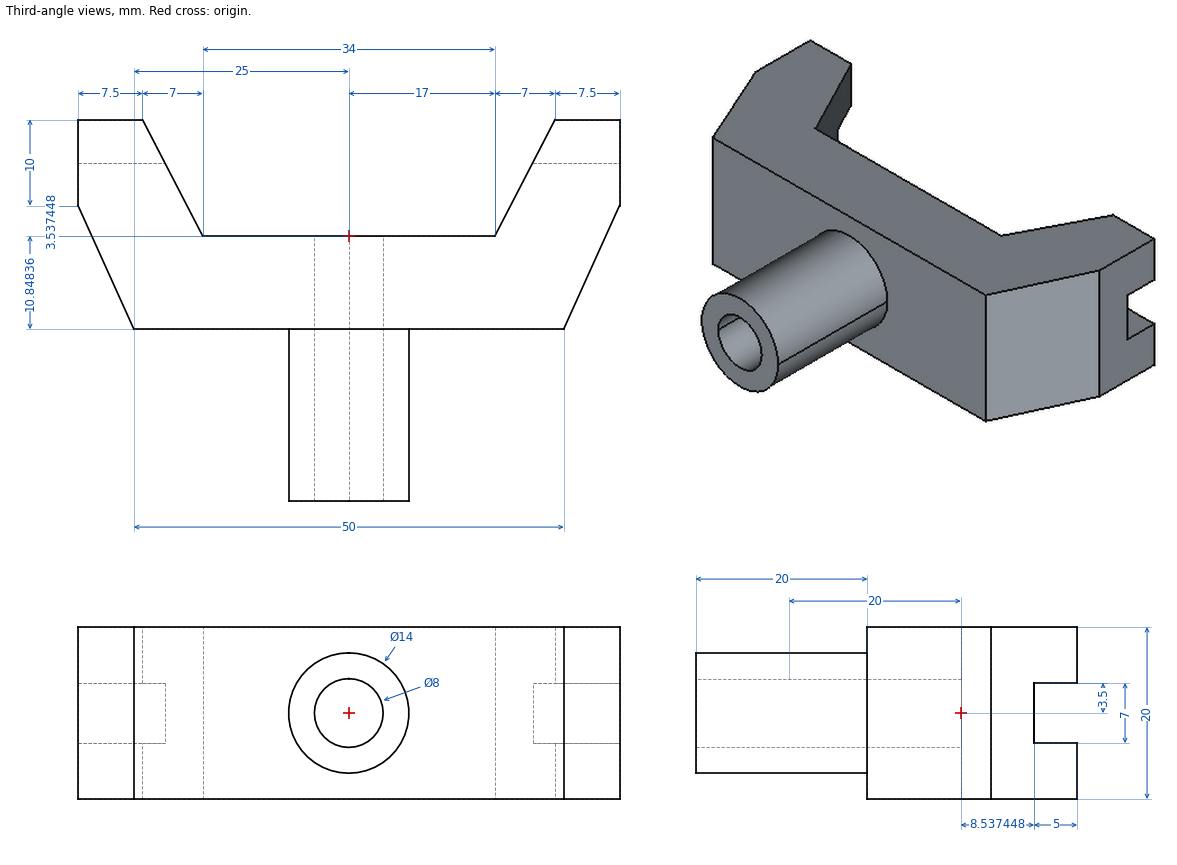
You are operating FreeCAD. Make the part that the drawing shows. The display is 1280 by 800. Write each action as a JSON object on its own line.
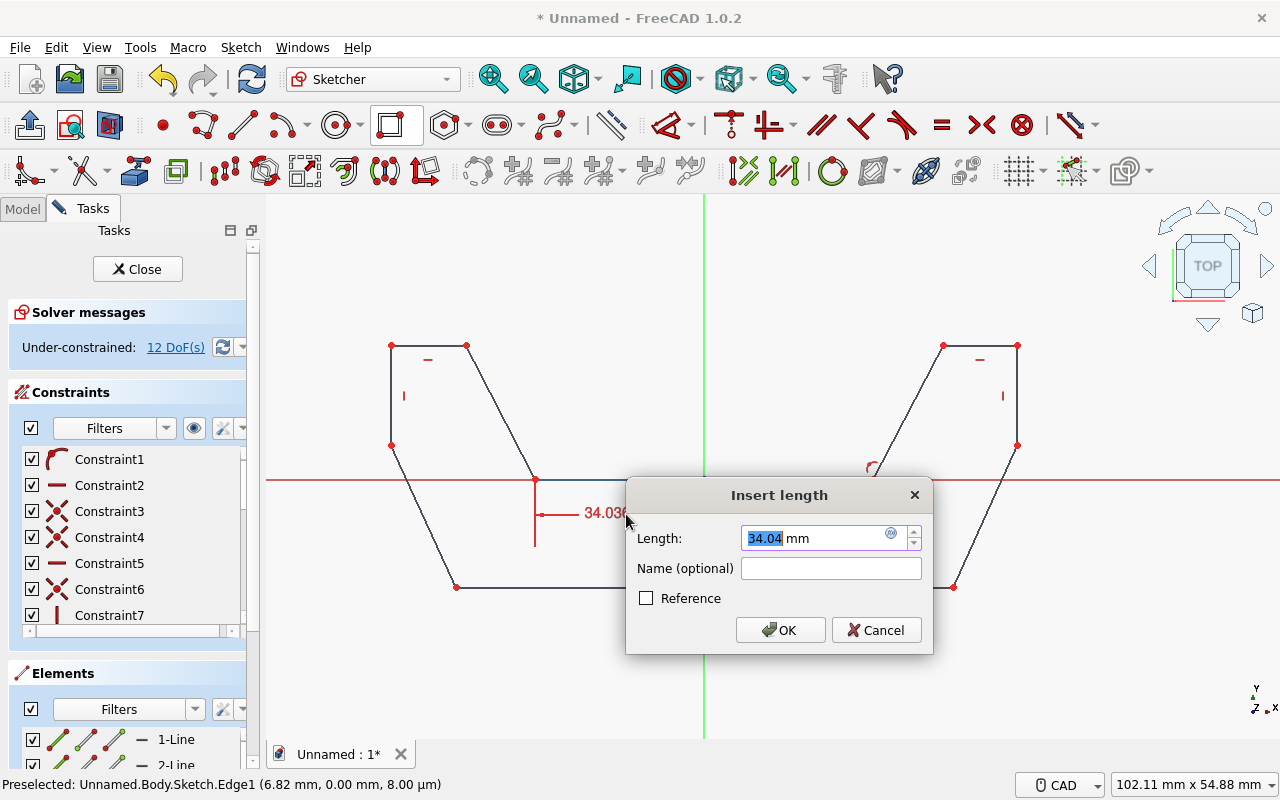
{"action": "type", "text": "34"}
{"action": "key", "text": "Return"}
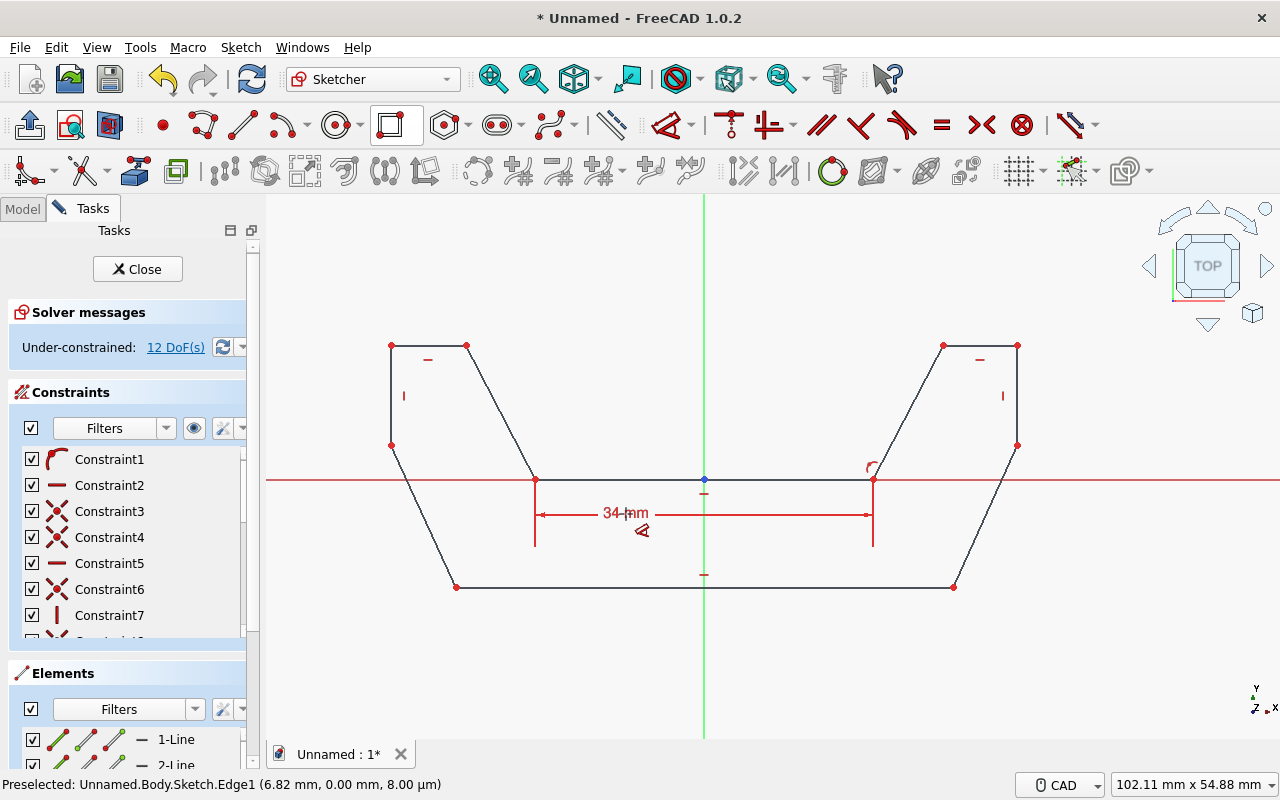
{"action": "left_click", "coordinate": [391, 376]}
{"action": "left_click", "coordinate": [357, 396]}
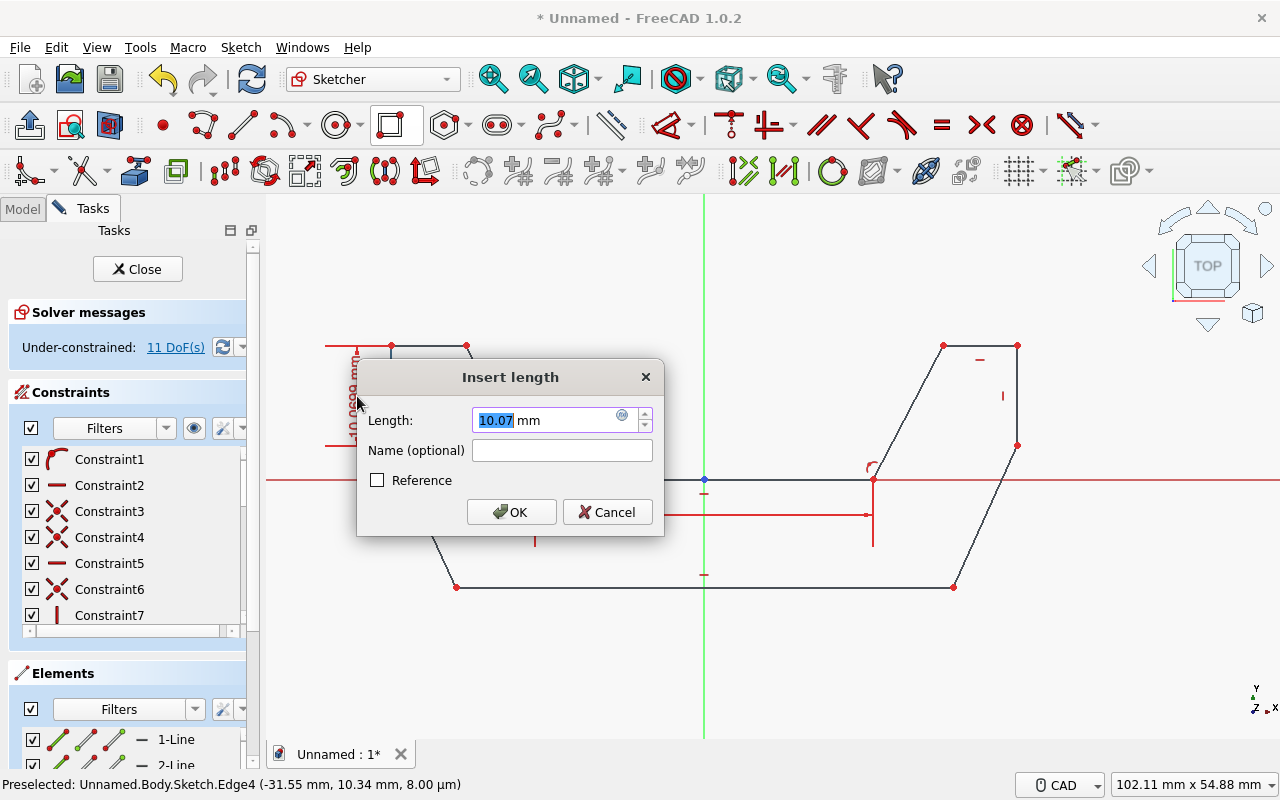
{"action": "type", "text": "10"}
{"action": "key", "text": "Return"}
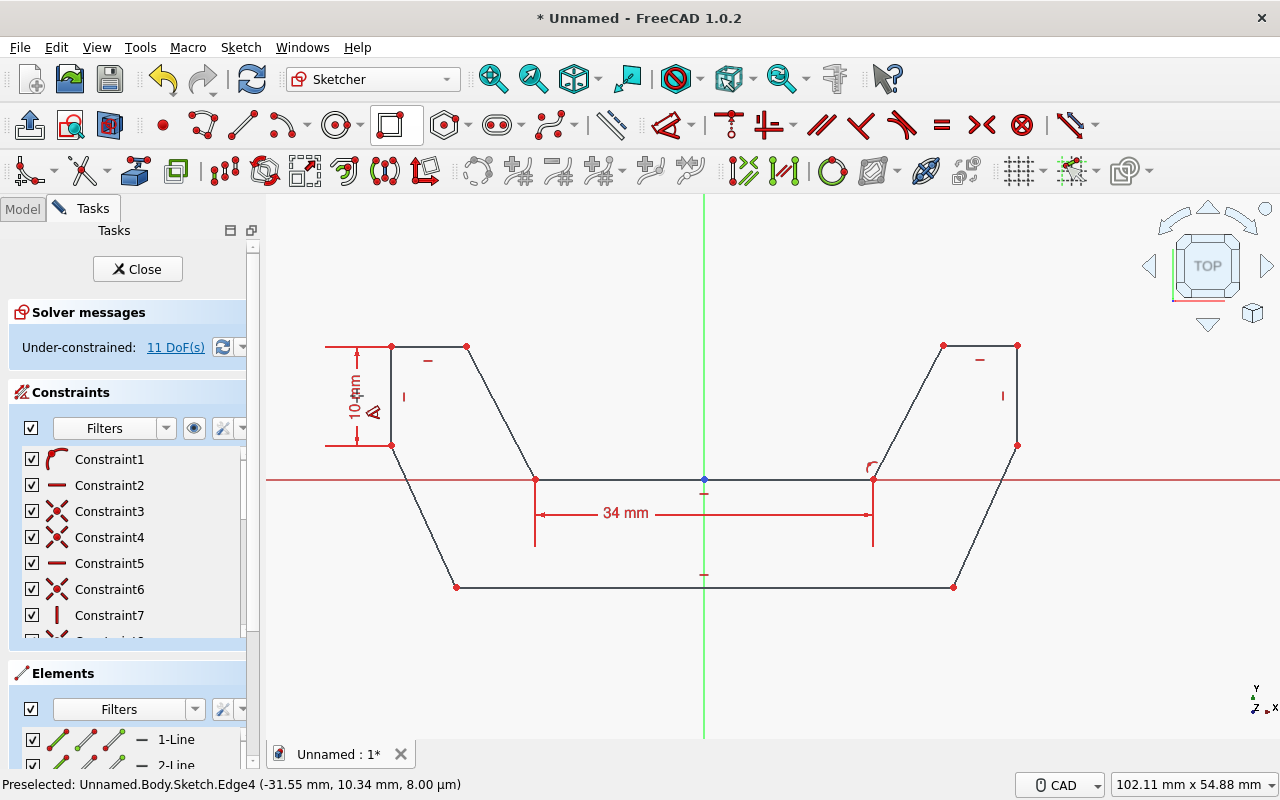
{"action": "left_click", "coordinate": [605, 588]}
{"action": "left_click", "coordinate": [590, 622]}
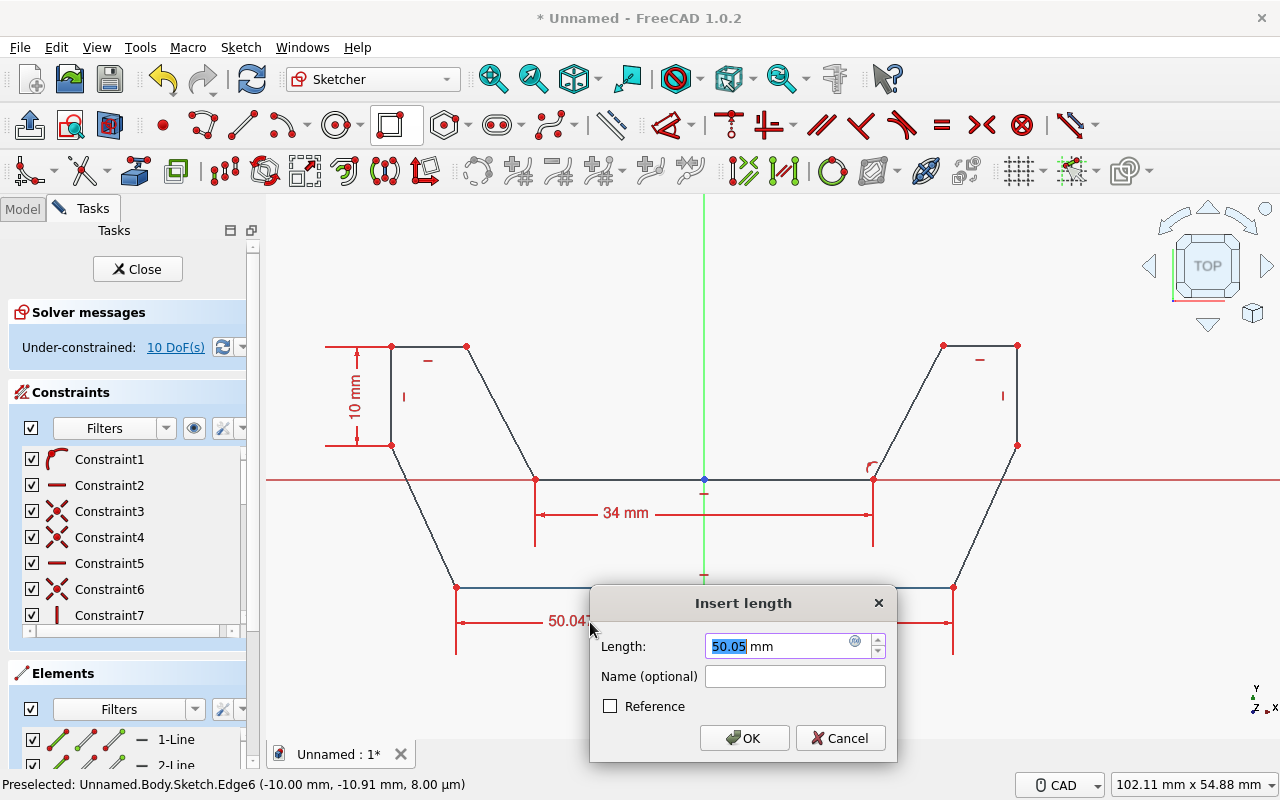
{"action": "type", "text": "50"}
{"action": "key", "text": "Return"}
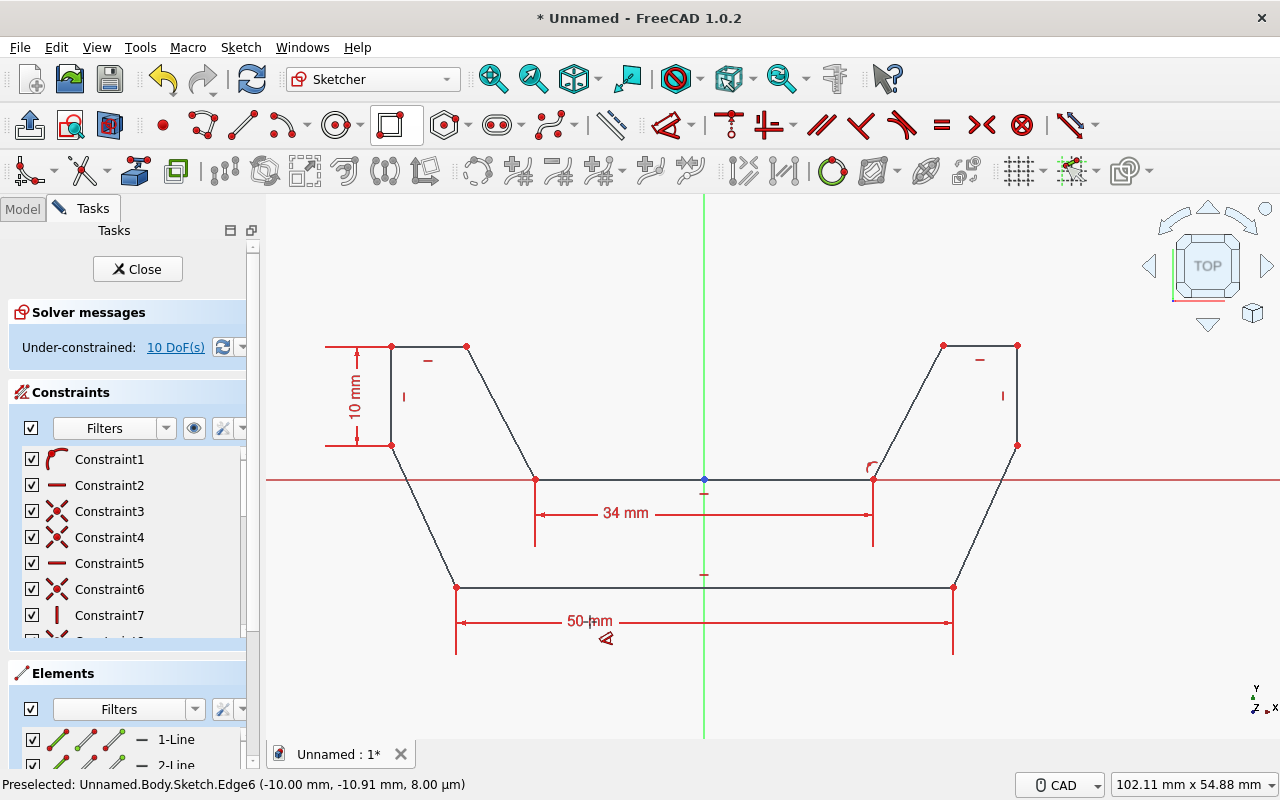
{"action": "left_click", "coordinate": [1017, 416]}
{"action": "left_click", "coordinate": [1051, 396]}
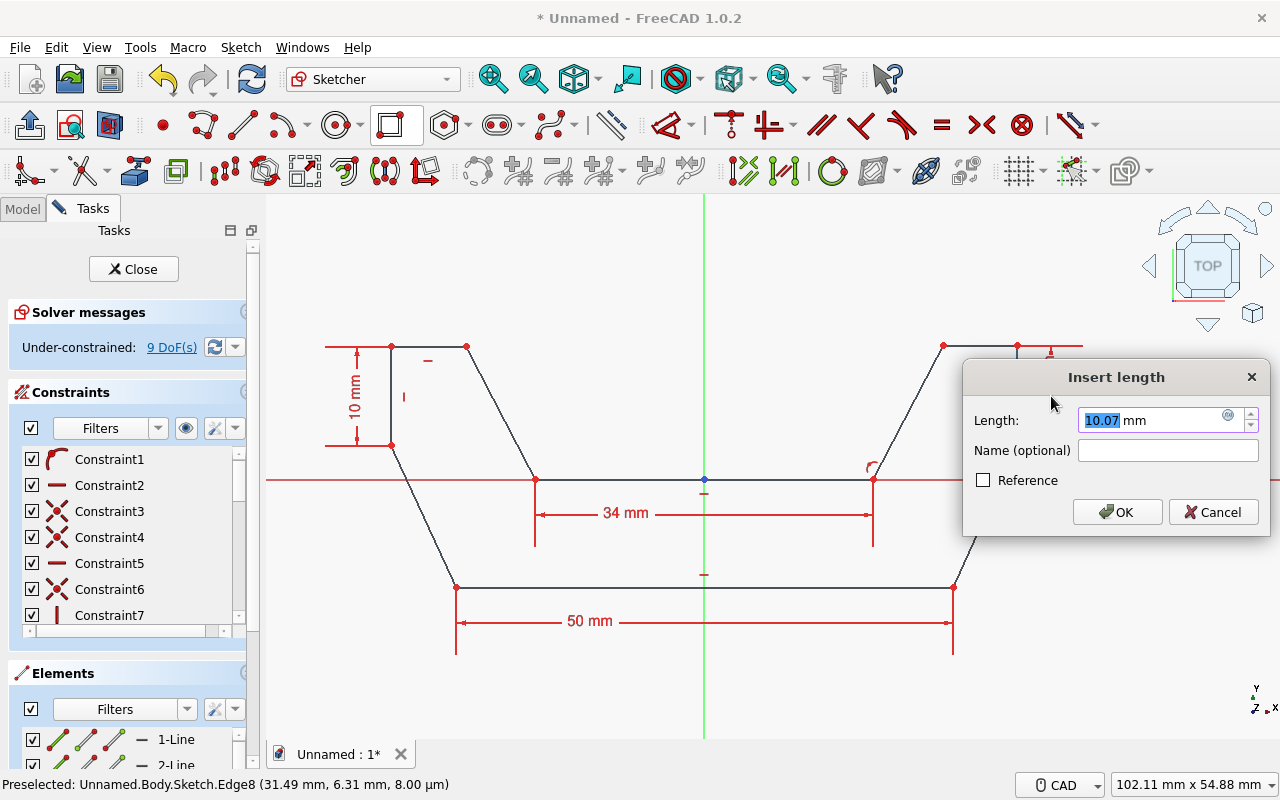
{"action": "type", "text": "10"}
{"action": "key", "text": "Return"}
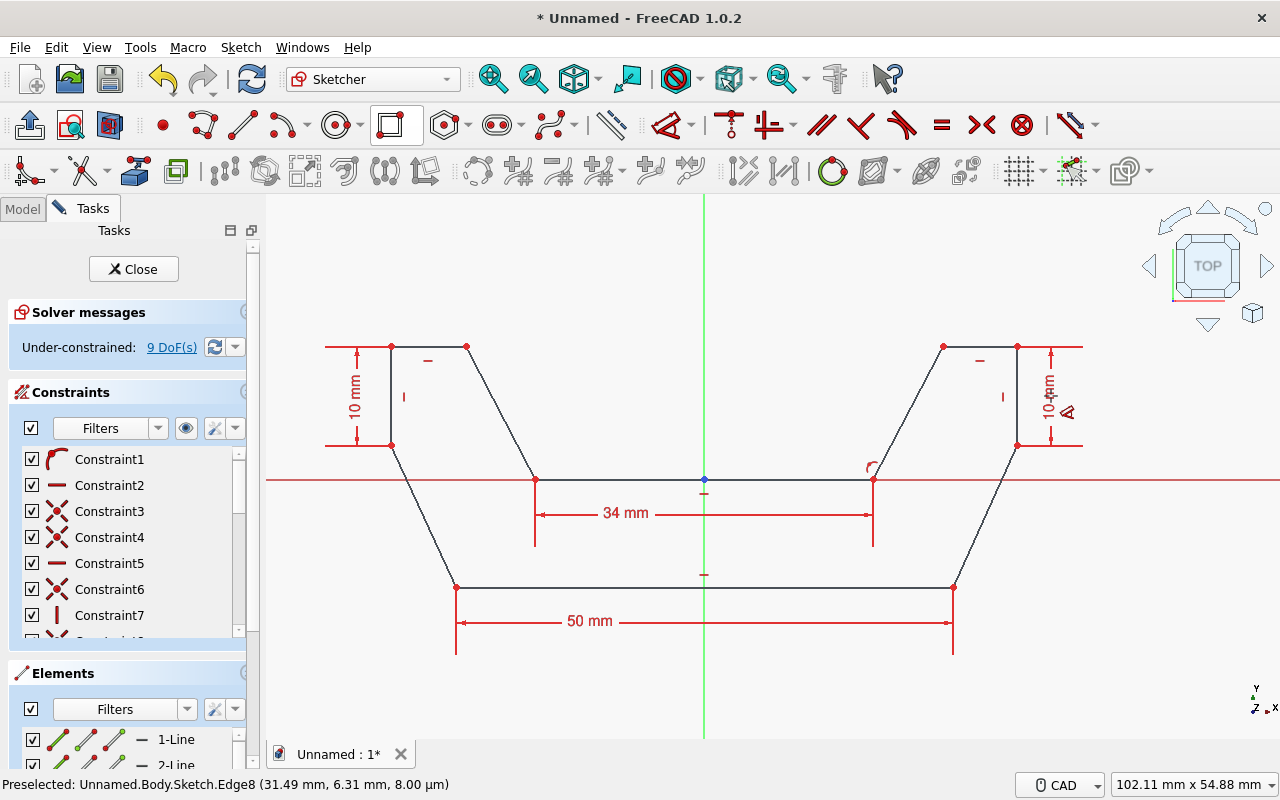
{"action": "left_click", "coordinate": [515, 440]}
{"action": "left_click", "coordinate": [501, 313]}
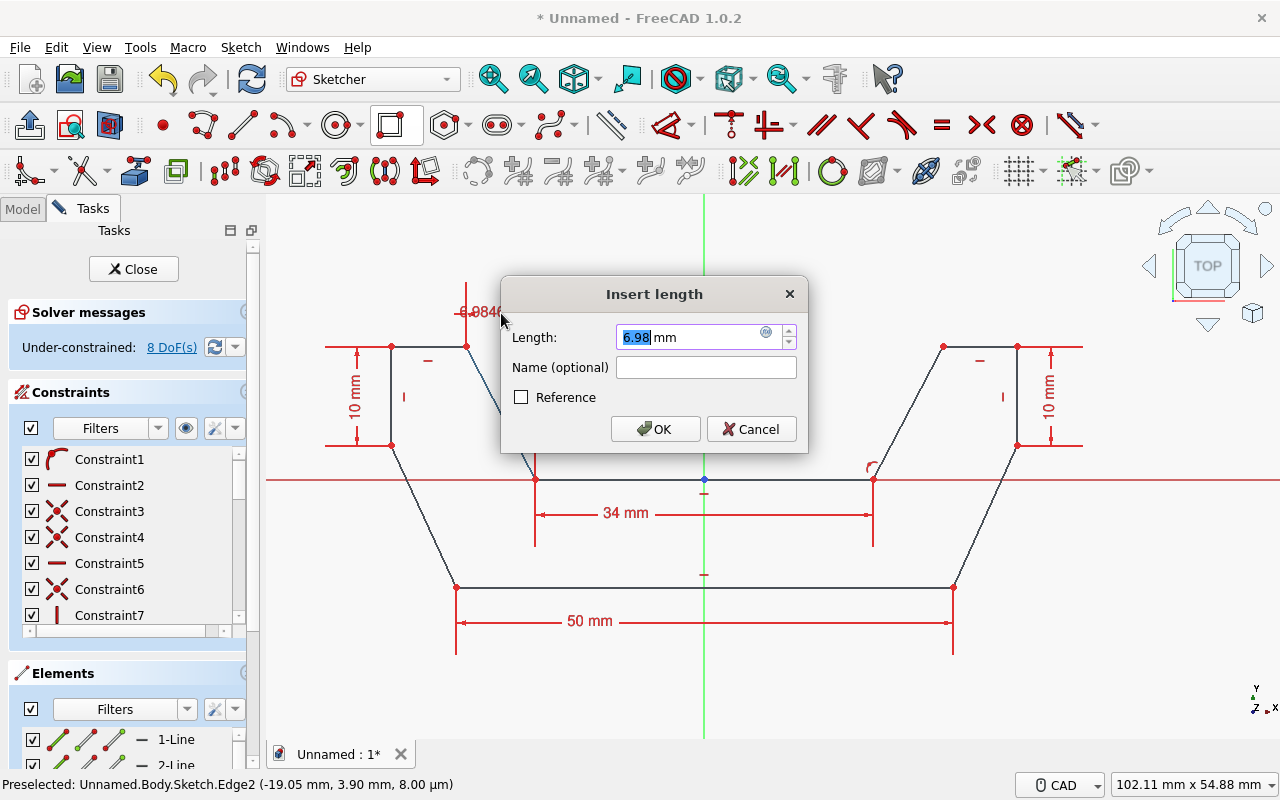
{"action": "type", "text": "7"}
{"action": "key", "text": "Return"}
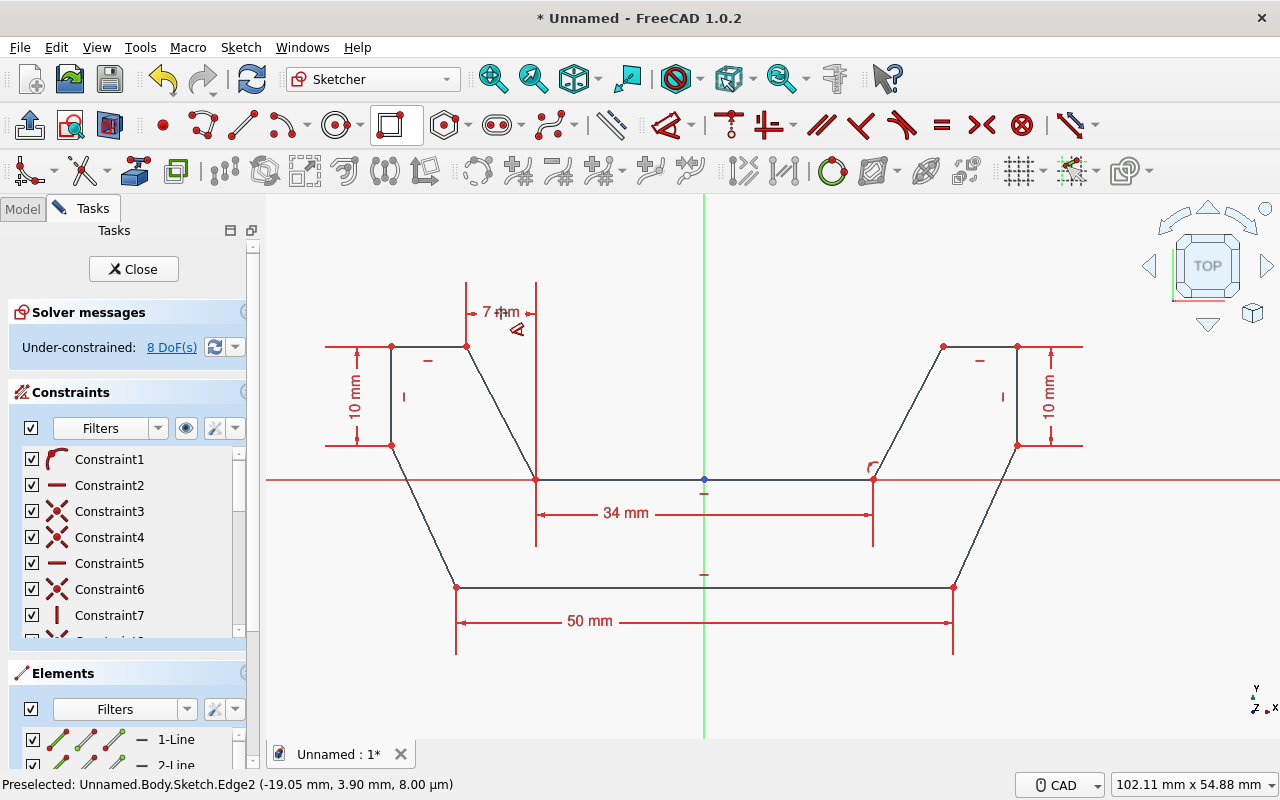
{"action": "left_click", "coordinate": [922, 387]}
{"action": "left_click", "coordinate": [908, 313]}